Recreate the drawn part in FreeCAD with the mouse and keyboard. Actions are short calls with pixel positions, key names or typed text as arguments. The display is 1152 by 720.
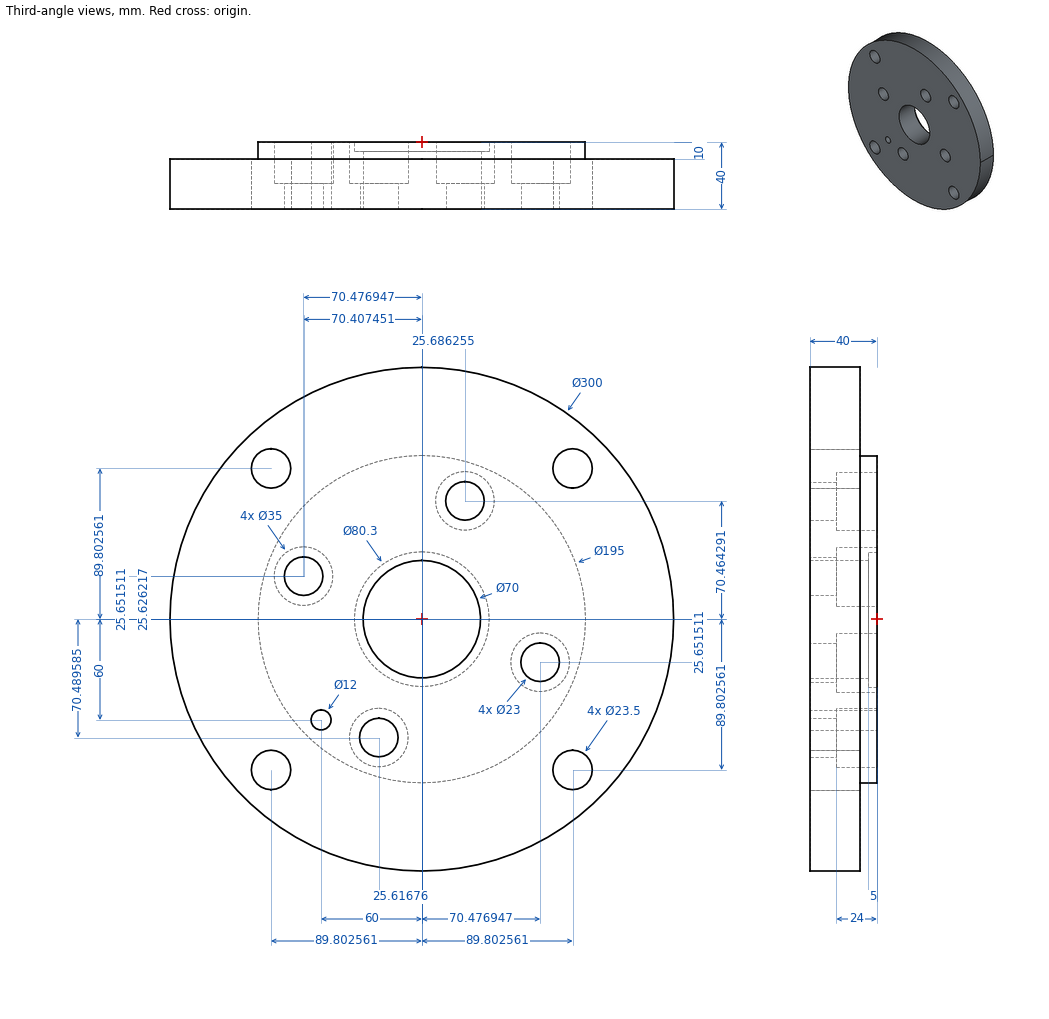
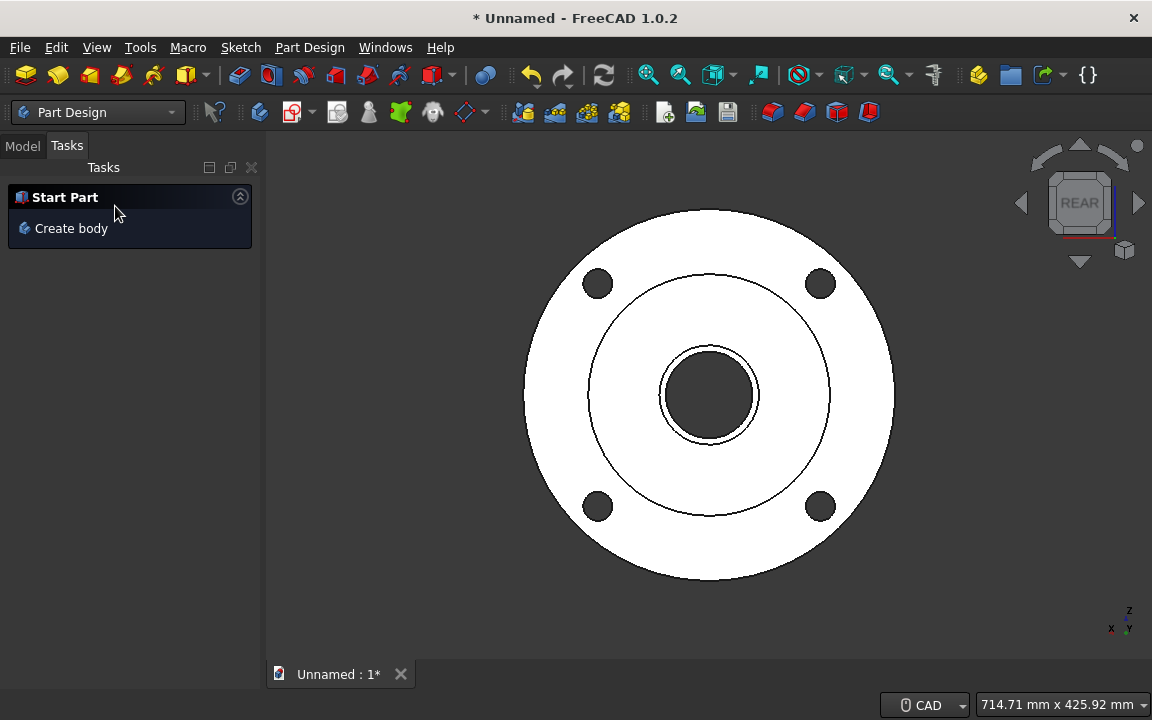
click(292, 112)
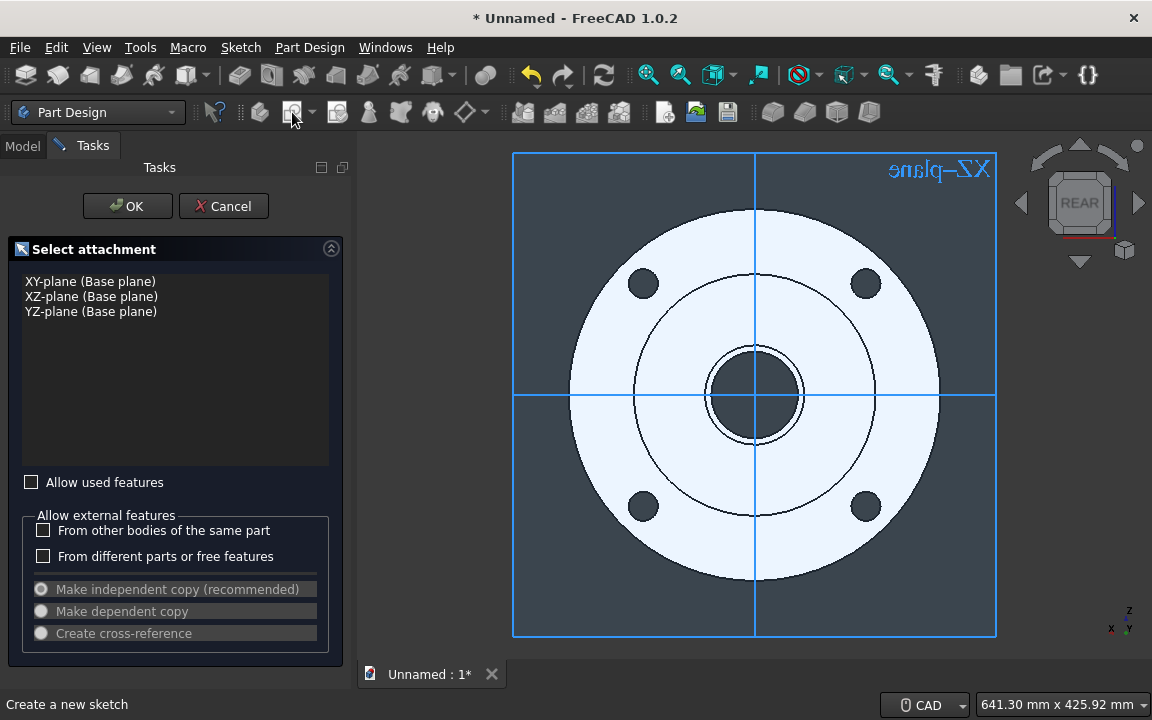
click(82, 296)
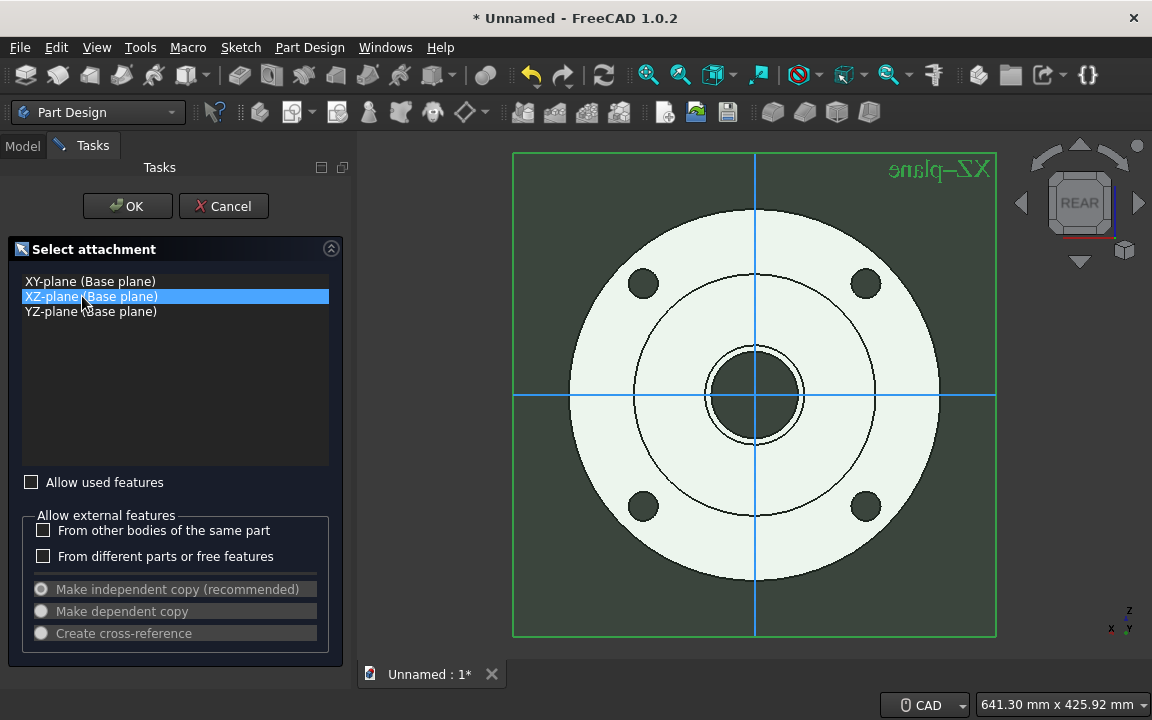
click(128, 206)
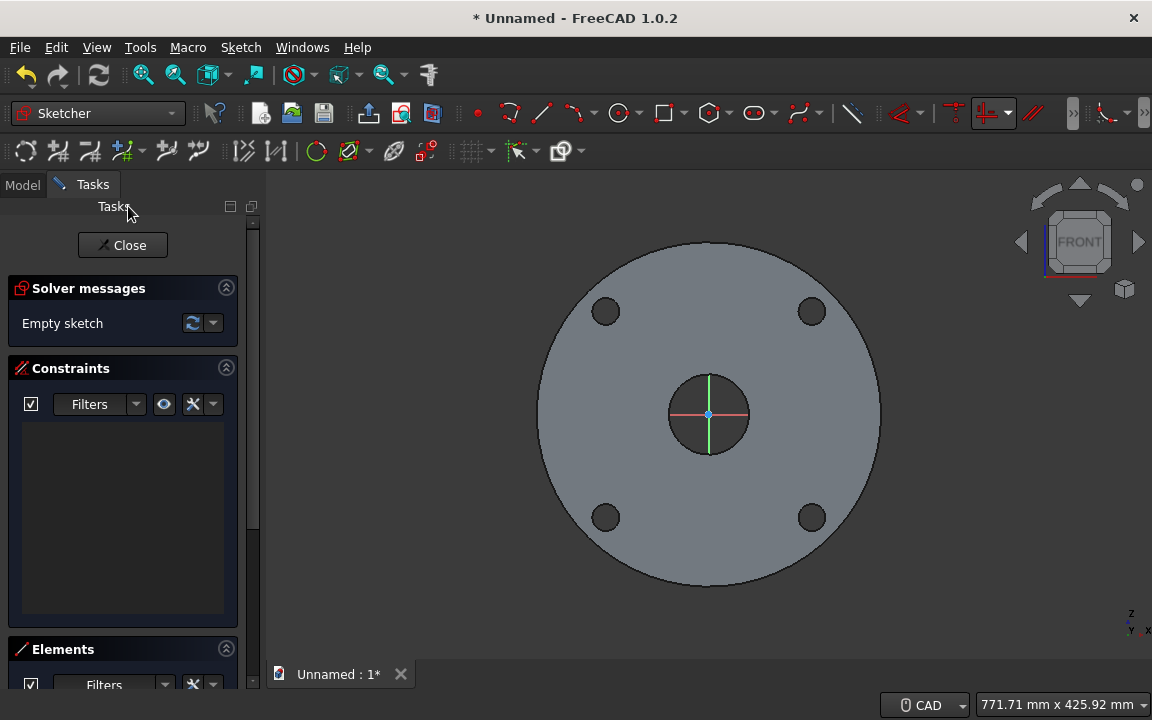
click(434, 114)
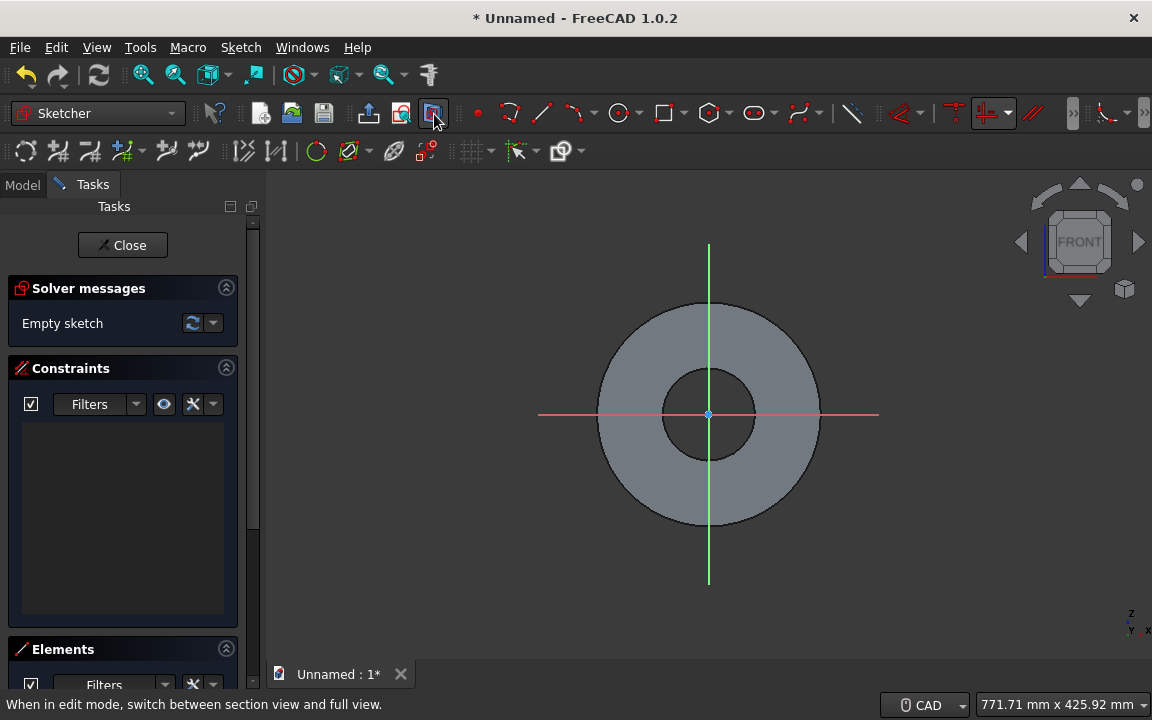
scroll(848, 415, up, 2)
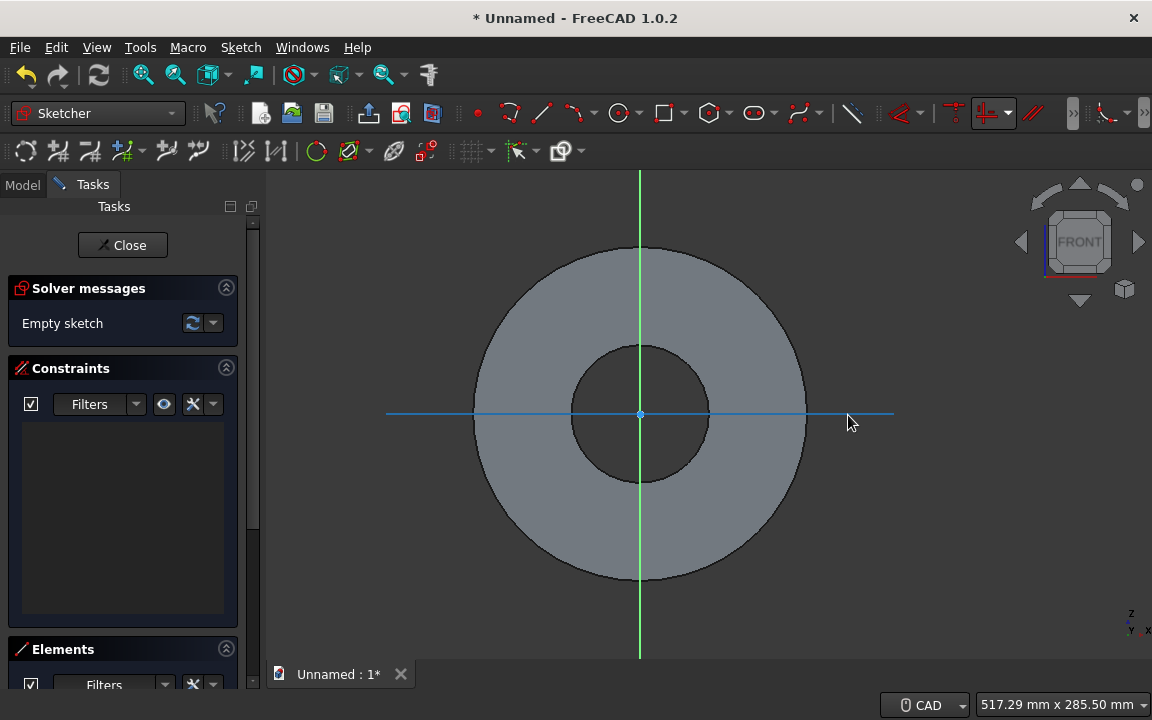
click(620, 114)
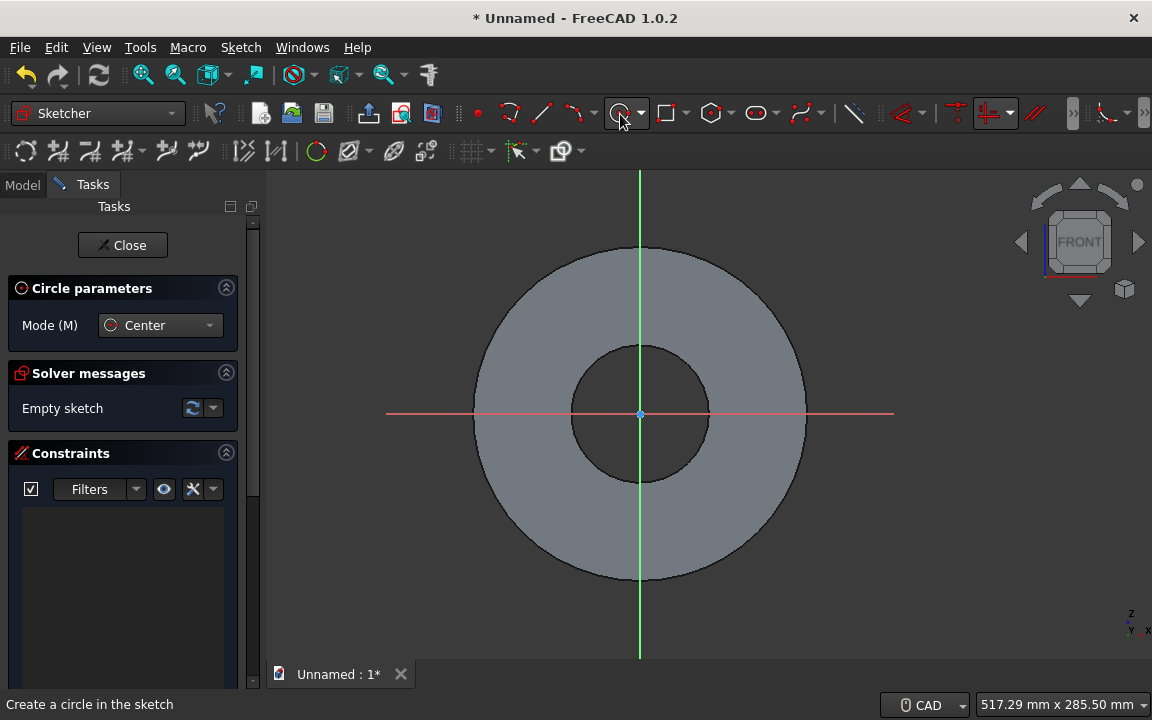
click(519, 370)
move(541, 349)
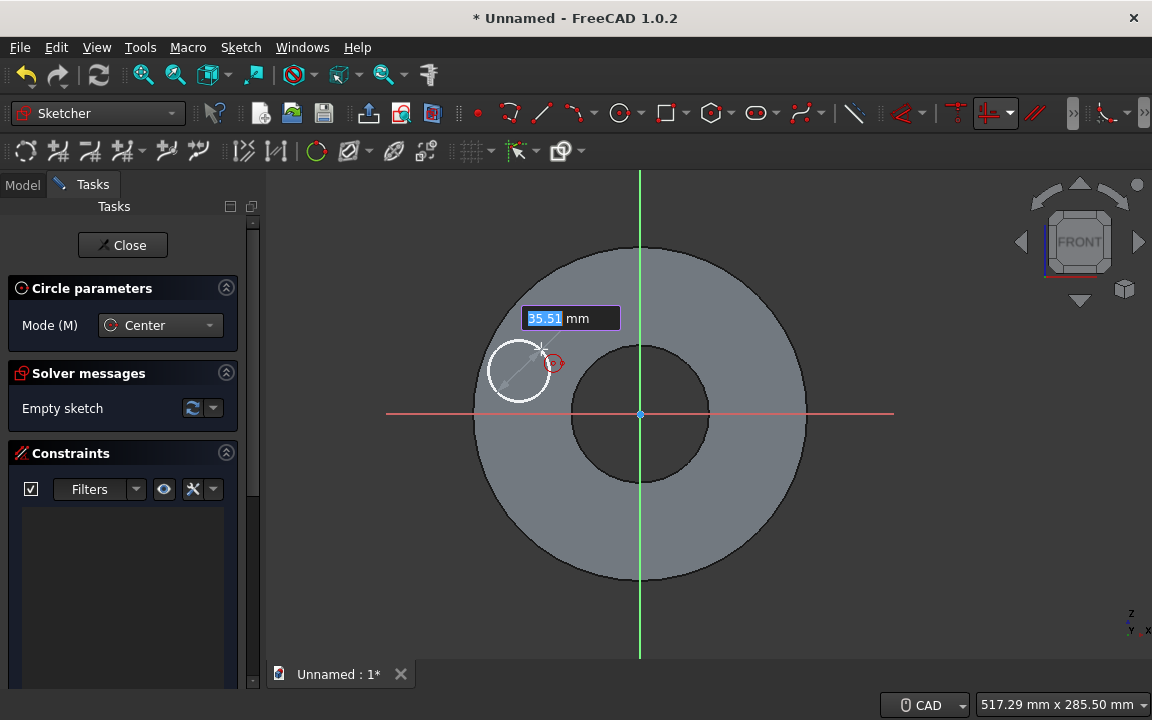
text(35)
key(Return)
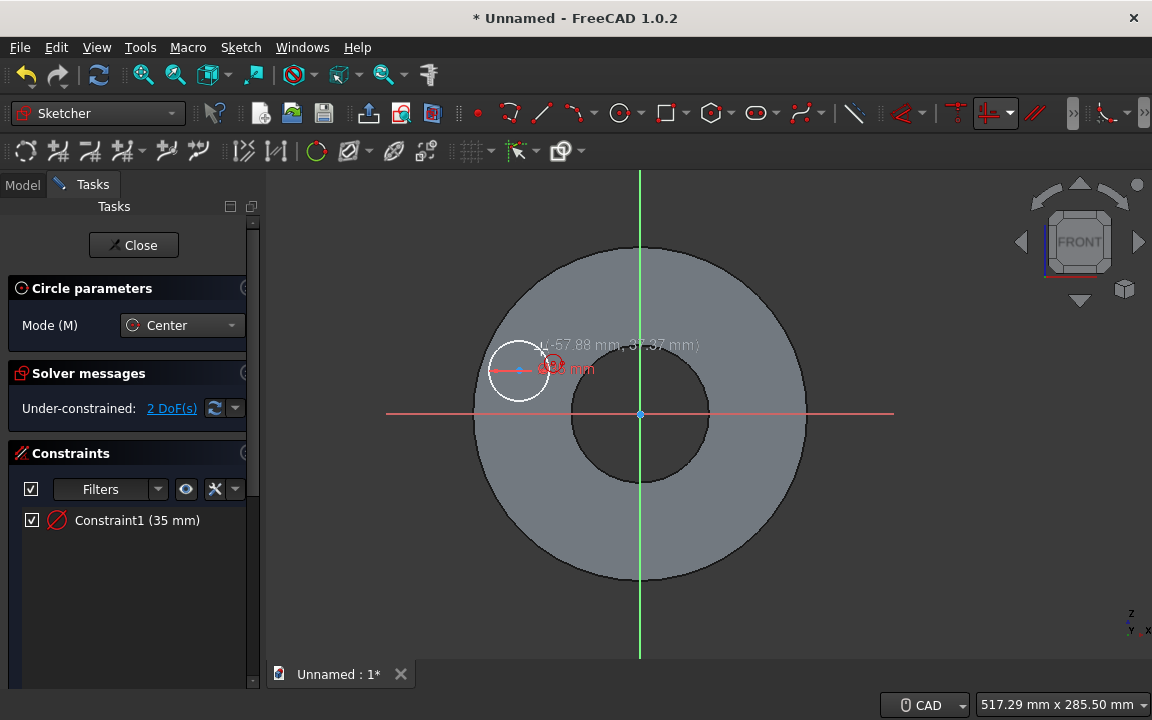
click(761, 458)
move(782, 437)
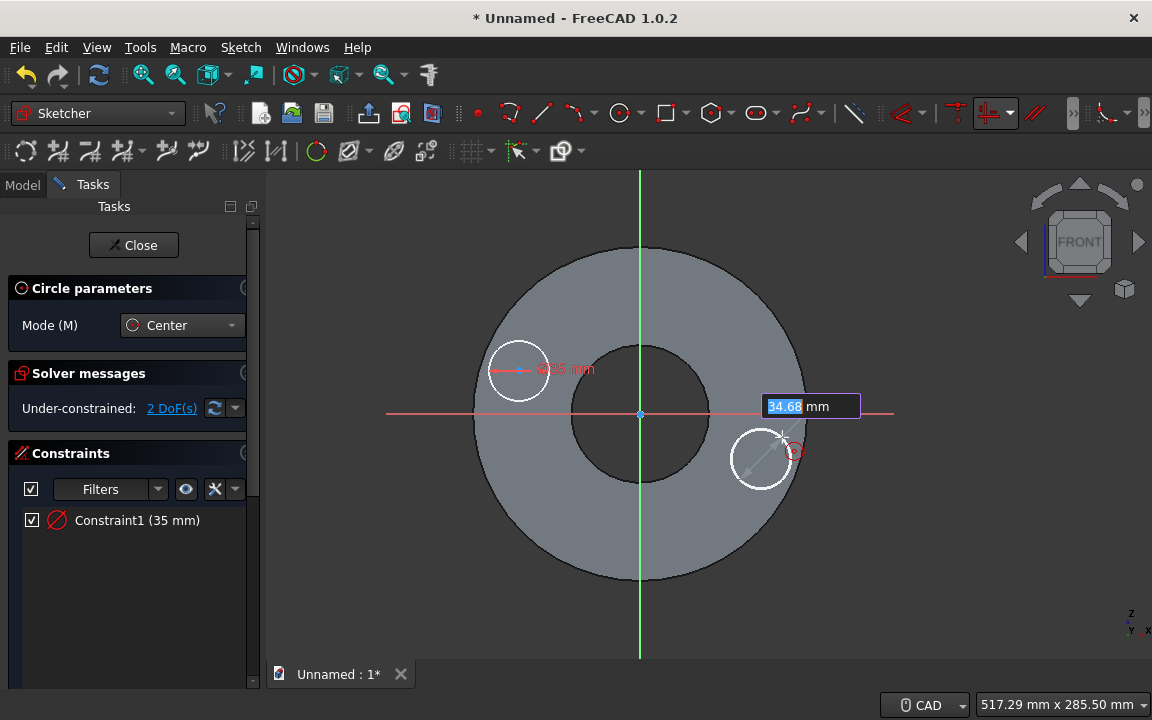
text(35)
key(Return)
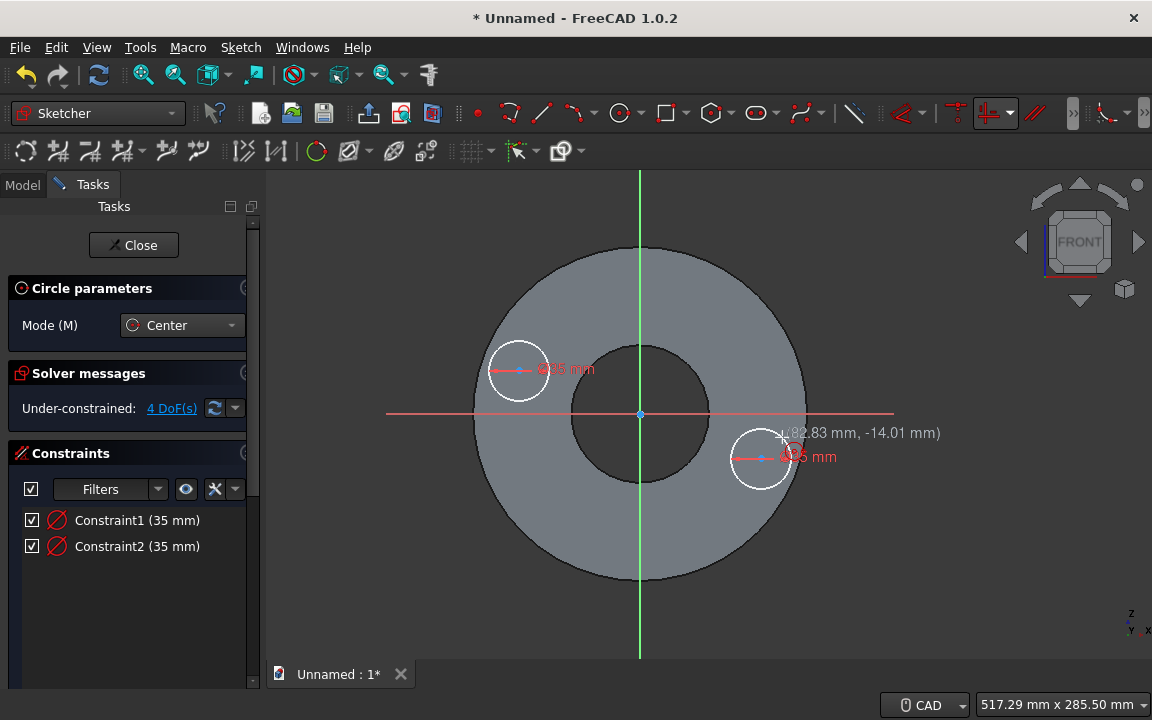
click(596, 535)
move(617, 514)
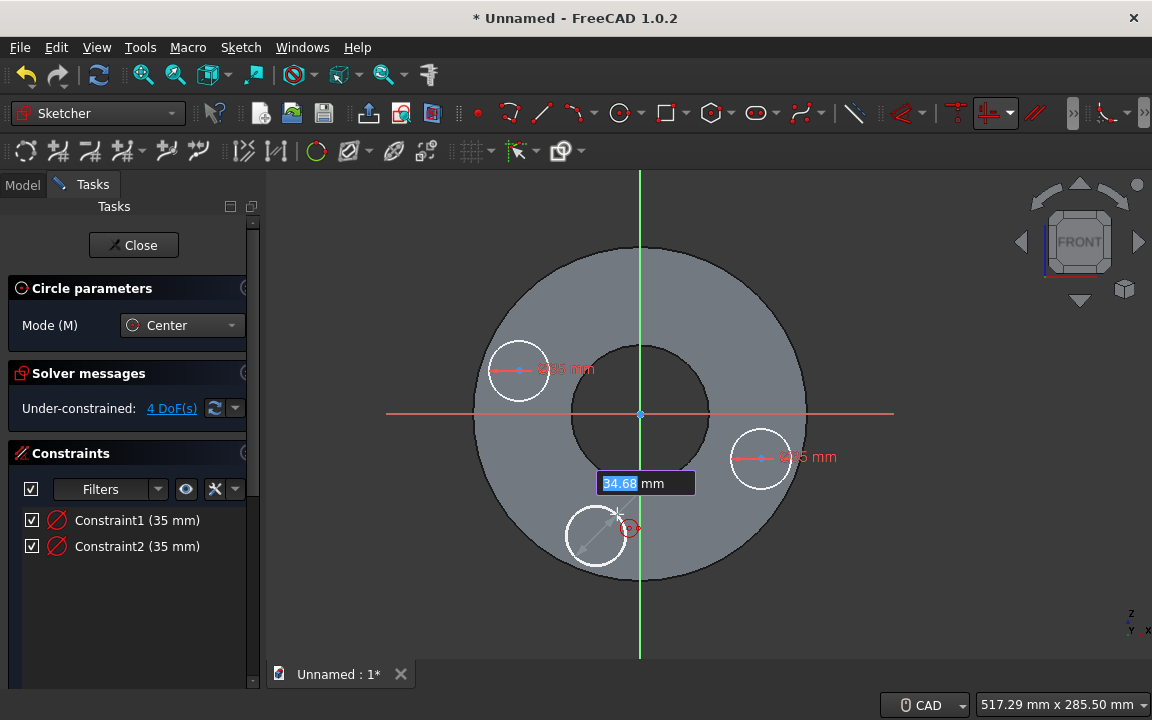
text(35)
key(Return)